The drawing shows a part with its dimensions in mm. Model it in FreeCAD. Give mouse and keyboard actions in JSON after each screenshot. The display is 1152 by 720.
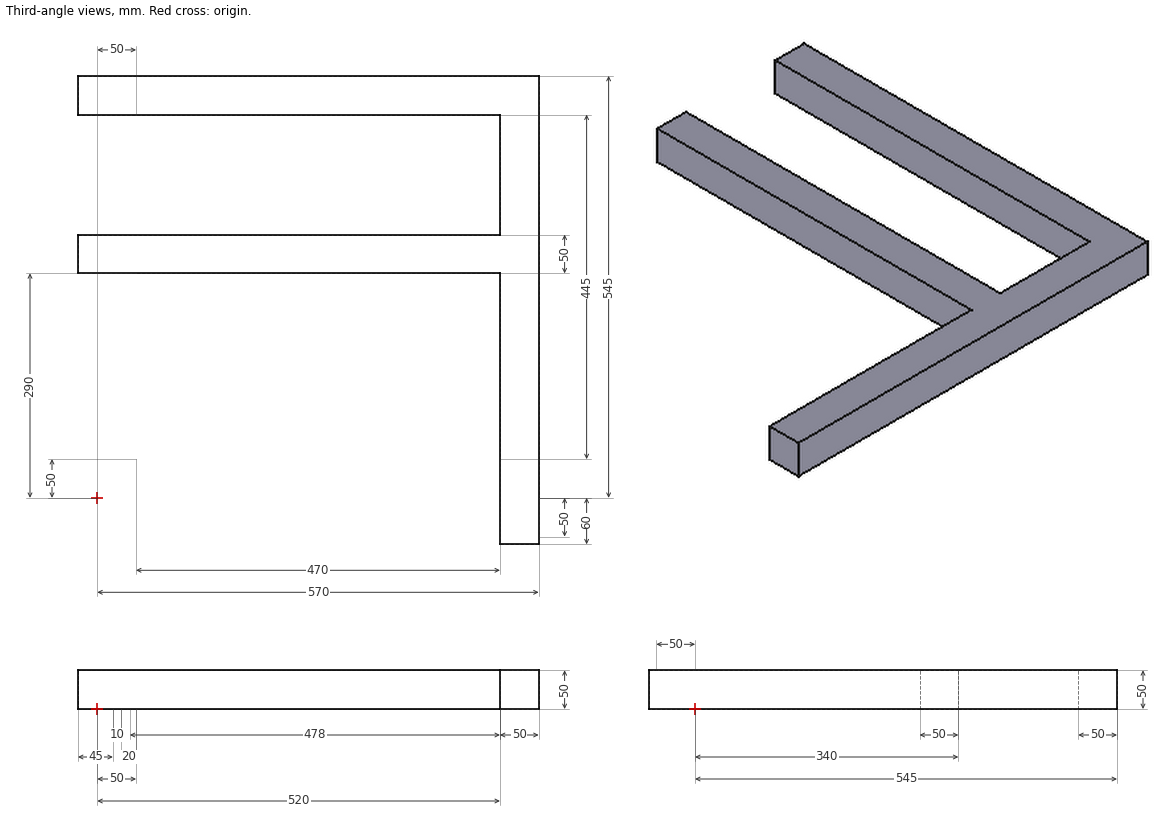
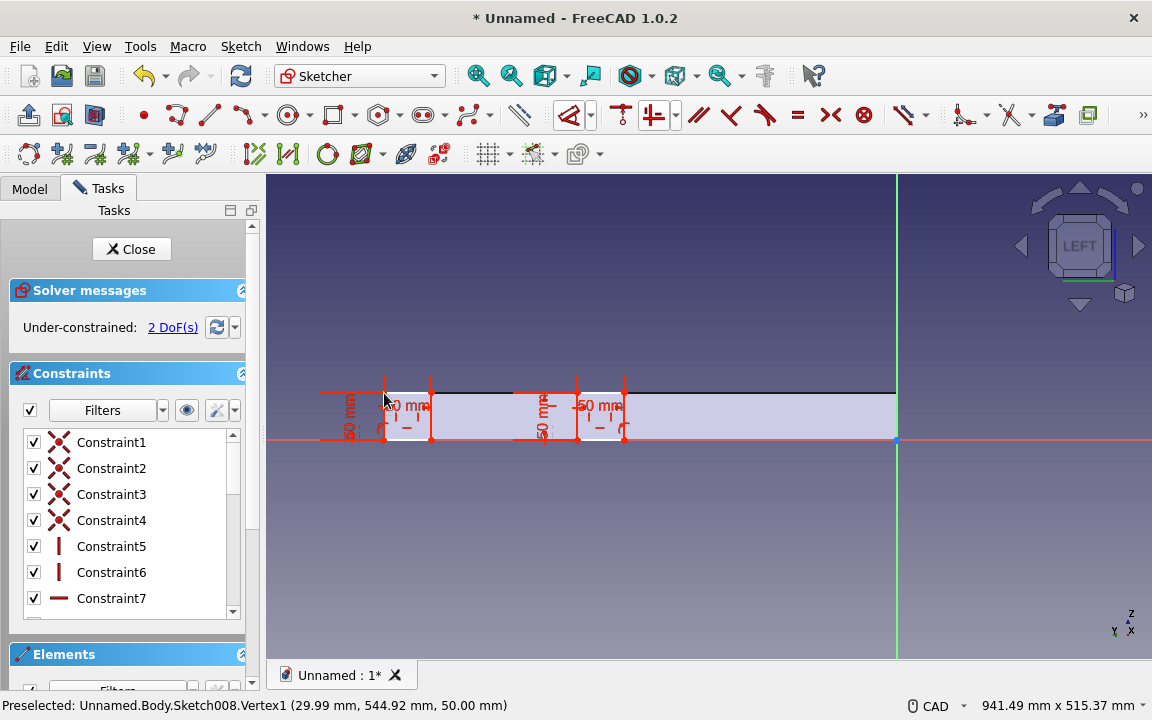
{"action": "key", "text": "l"}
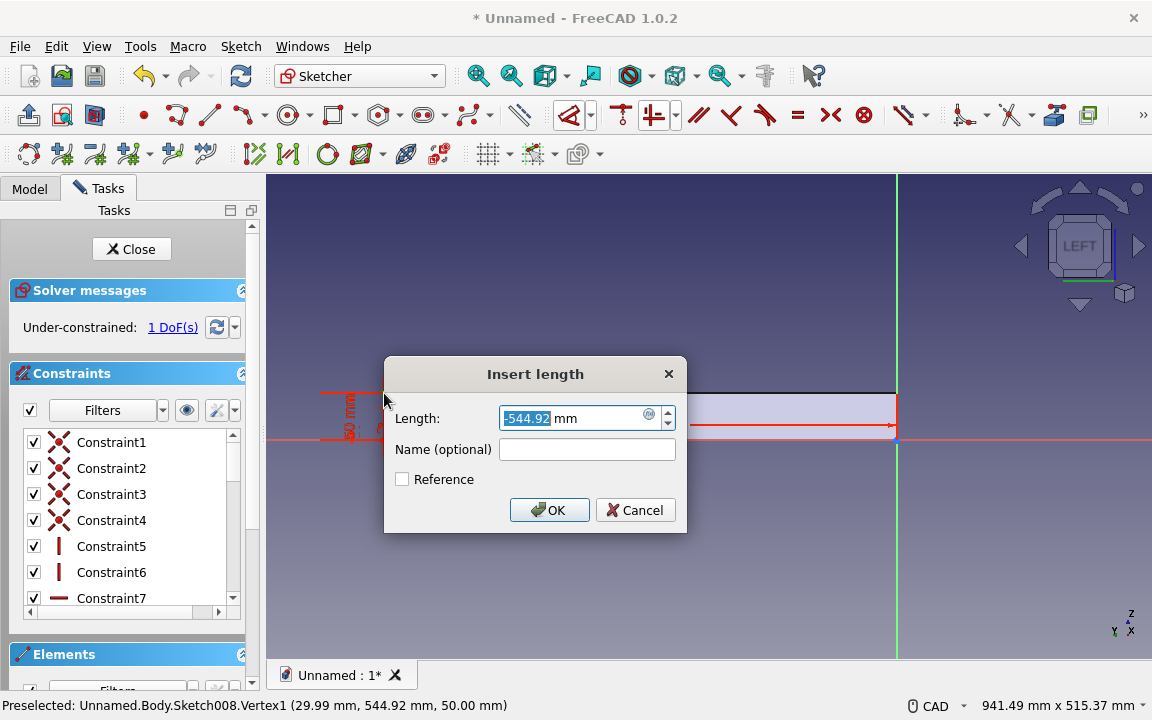
{"action": "type", "text": "-545"}
{"action": "key", "text": "Return"}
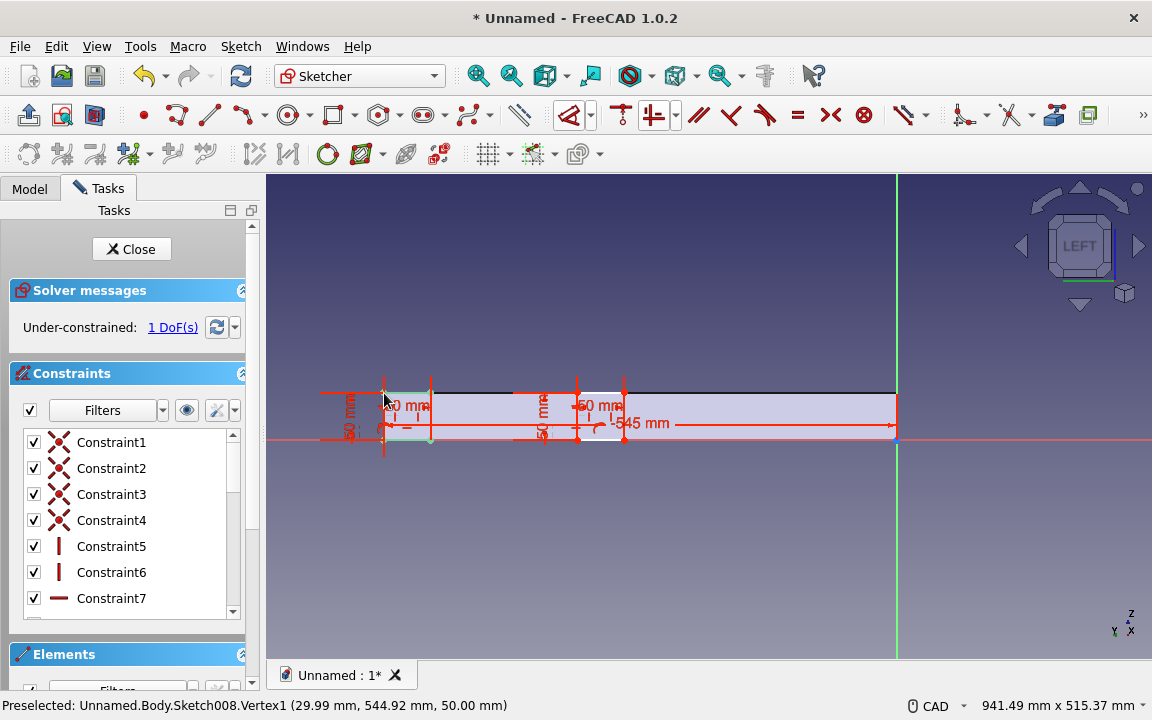
{"action": "left_click", "coordinate": [577, 393]}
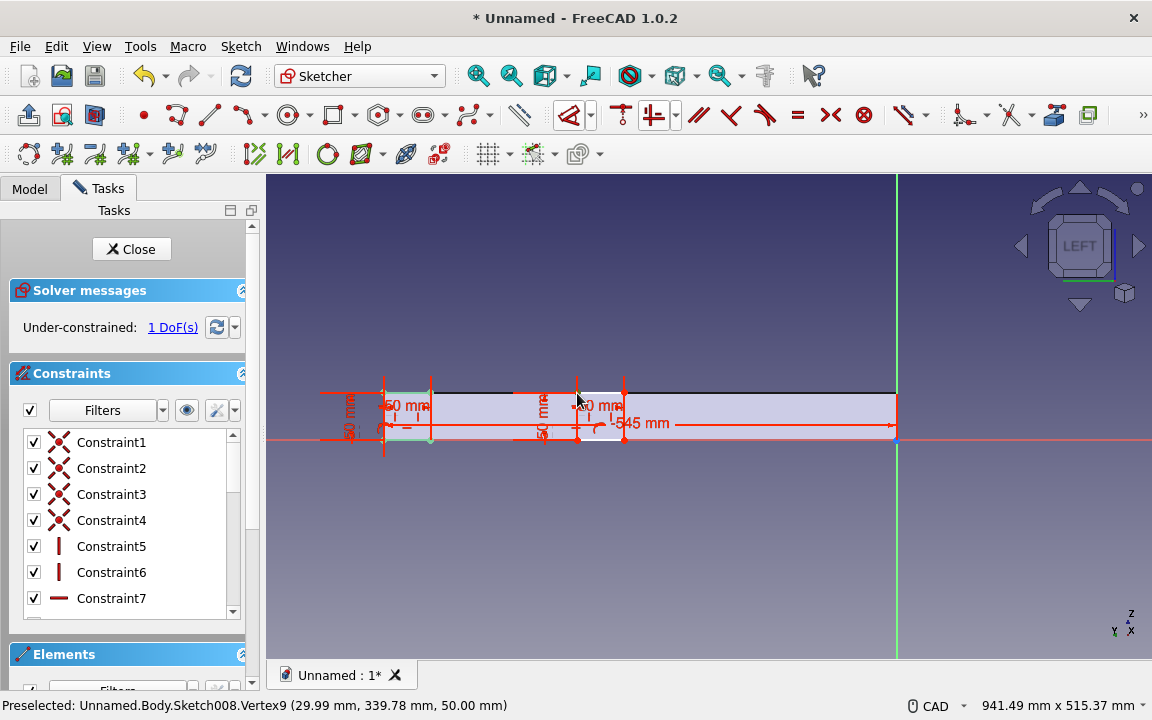
{"action": "key", "text": "l"}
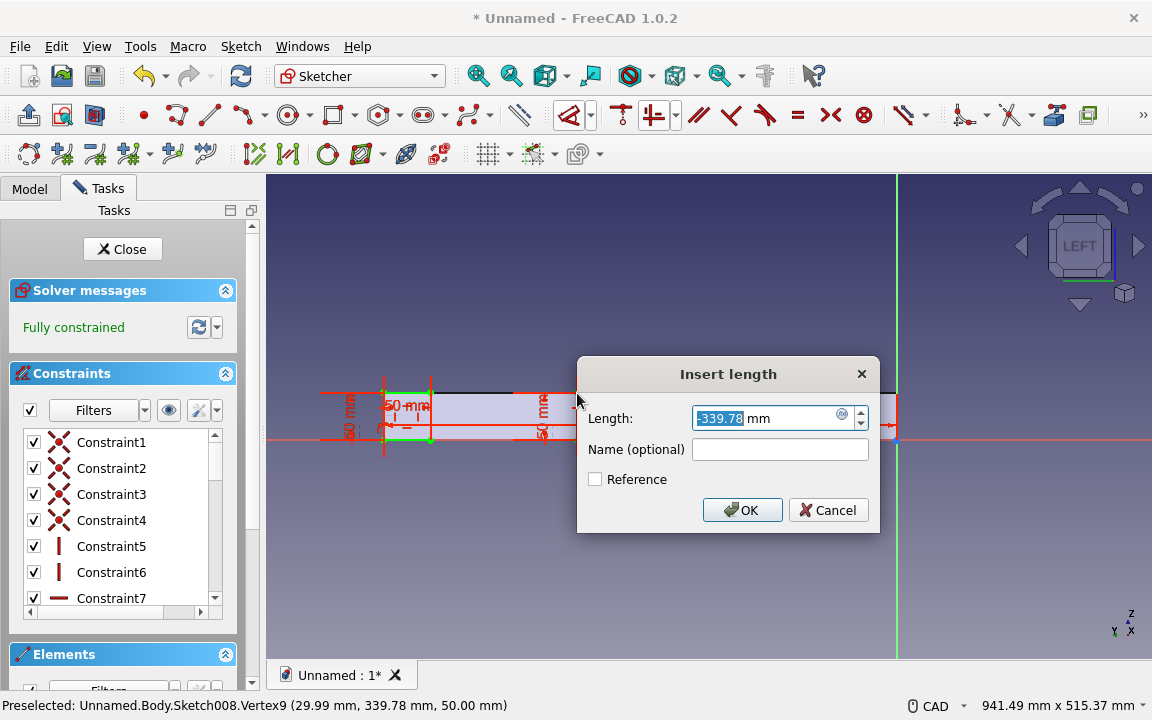
{"action": "type", "text": "-340"}
{"action": "key", "text": "Return"}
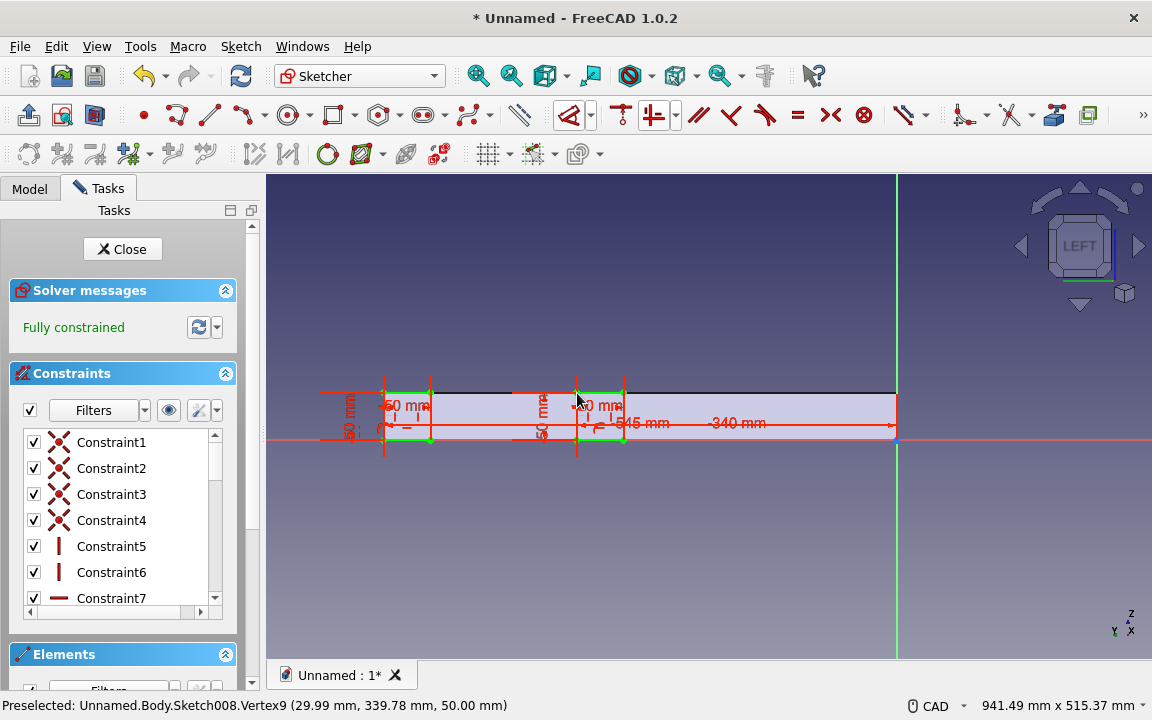
{"action": "left_click", "coordinate": [123, 249]}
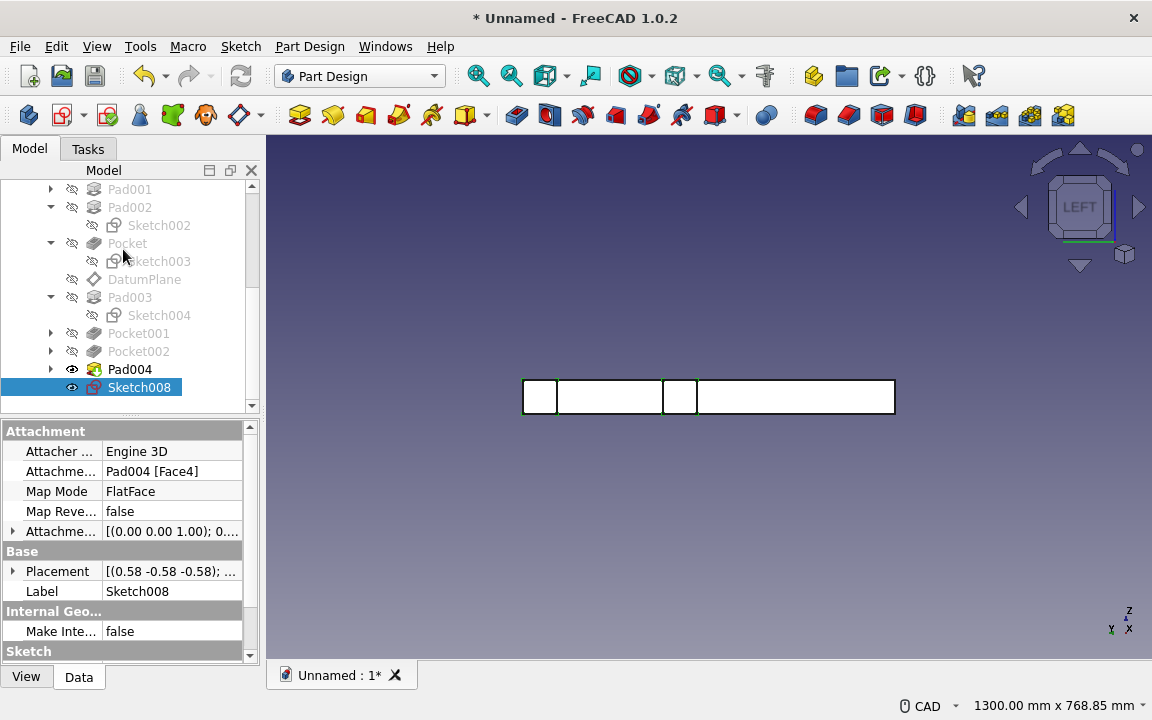
{"action": "left_click", "coordinate": [300, 116]}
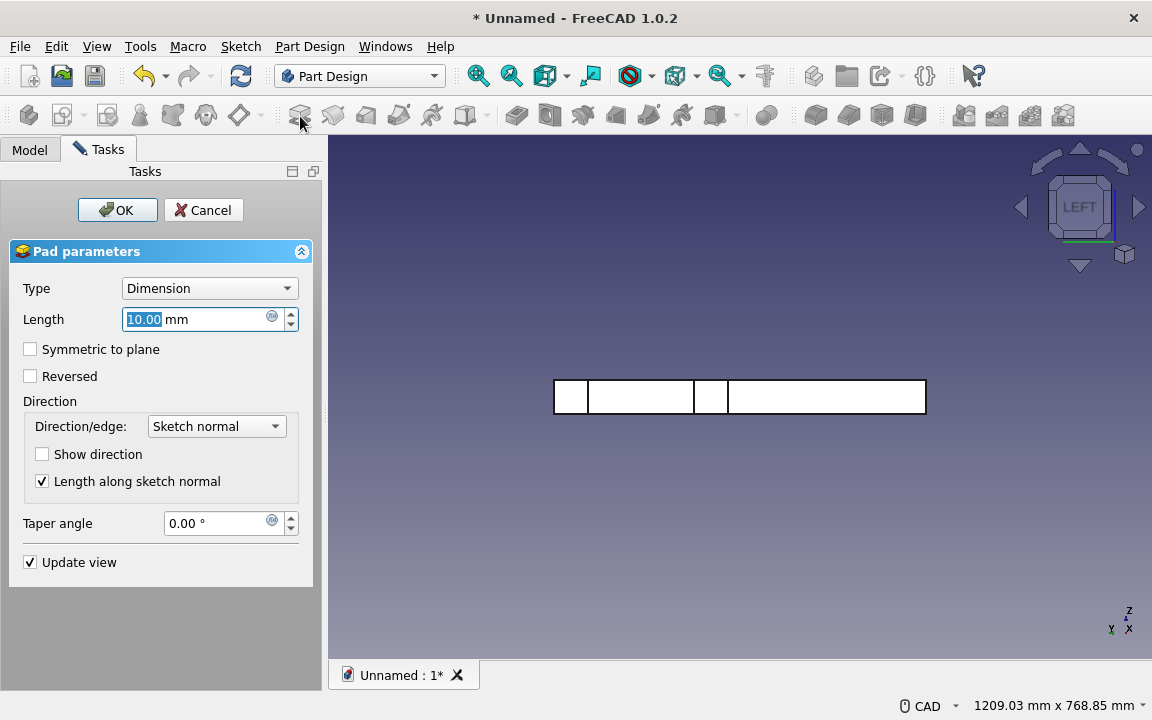
{"action": "type", "text": "10"}
{"action": "key", "text": "Tab"}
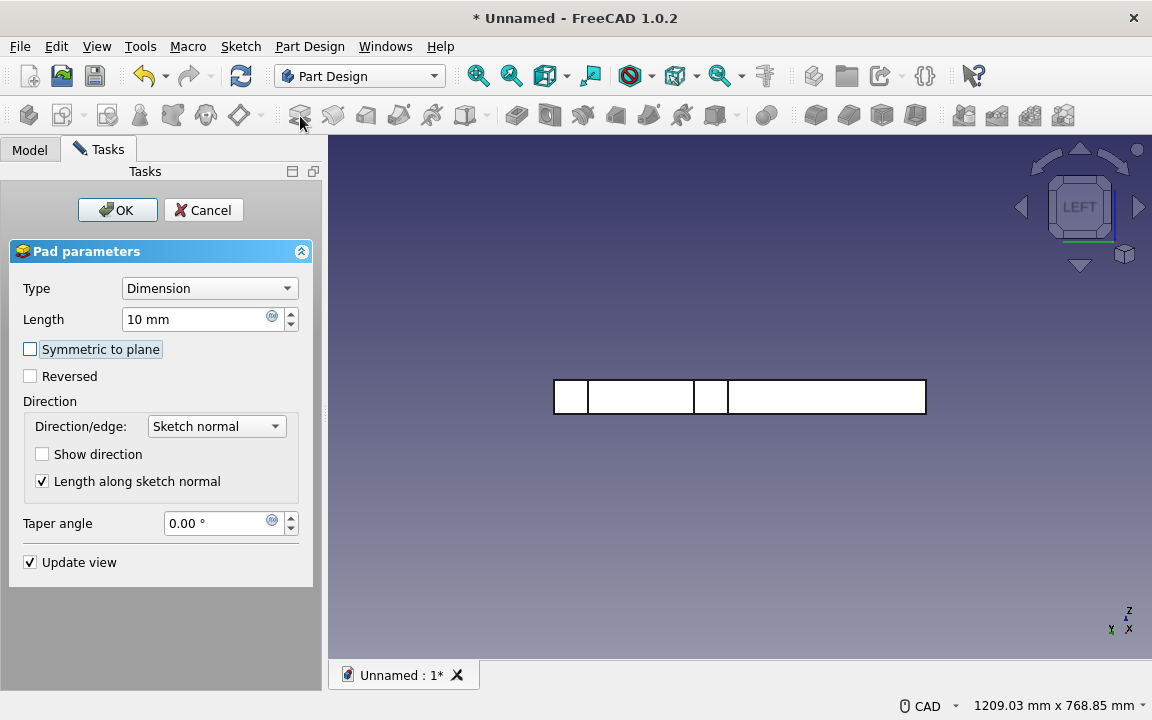
{"action": "left_click", "coordinate": [118, 210]}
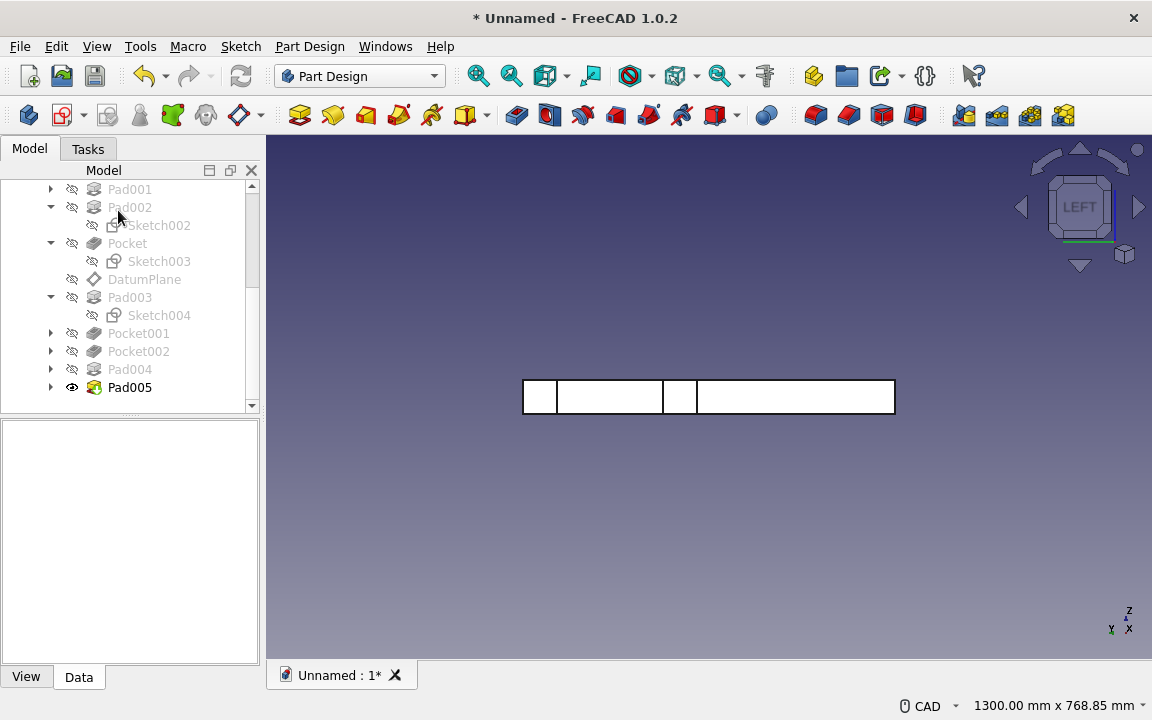
{"action": "key", "text": "v f"}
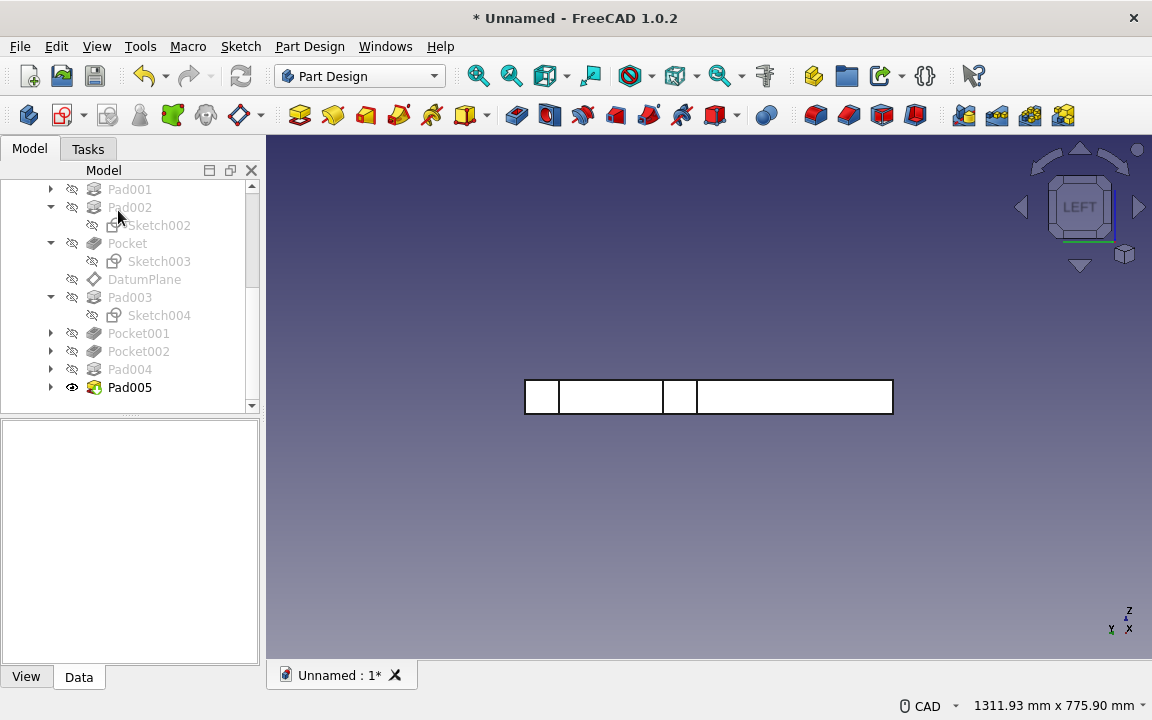
{"action": "key", "text": "0"}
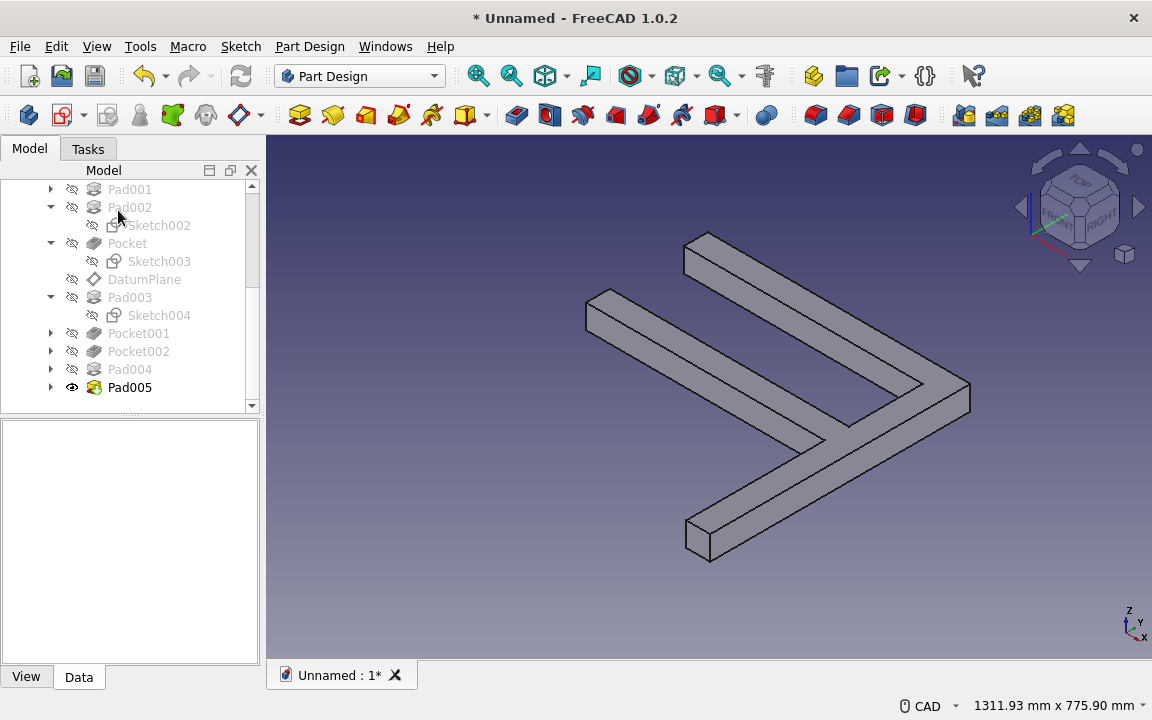
{"action": "left_click", "coordinate": [698, 540]}